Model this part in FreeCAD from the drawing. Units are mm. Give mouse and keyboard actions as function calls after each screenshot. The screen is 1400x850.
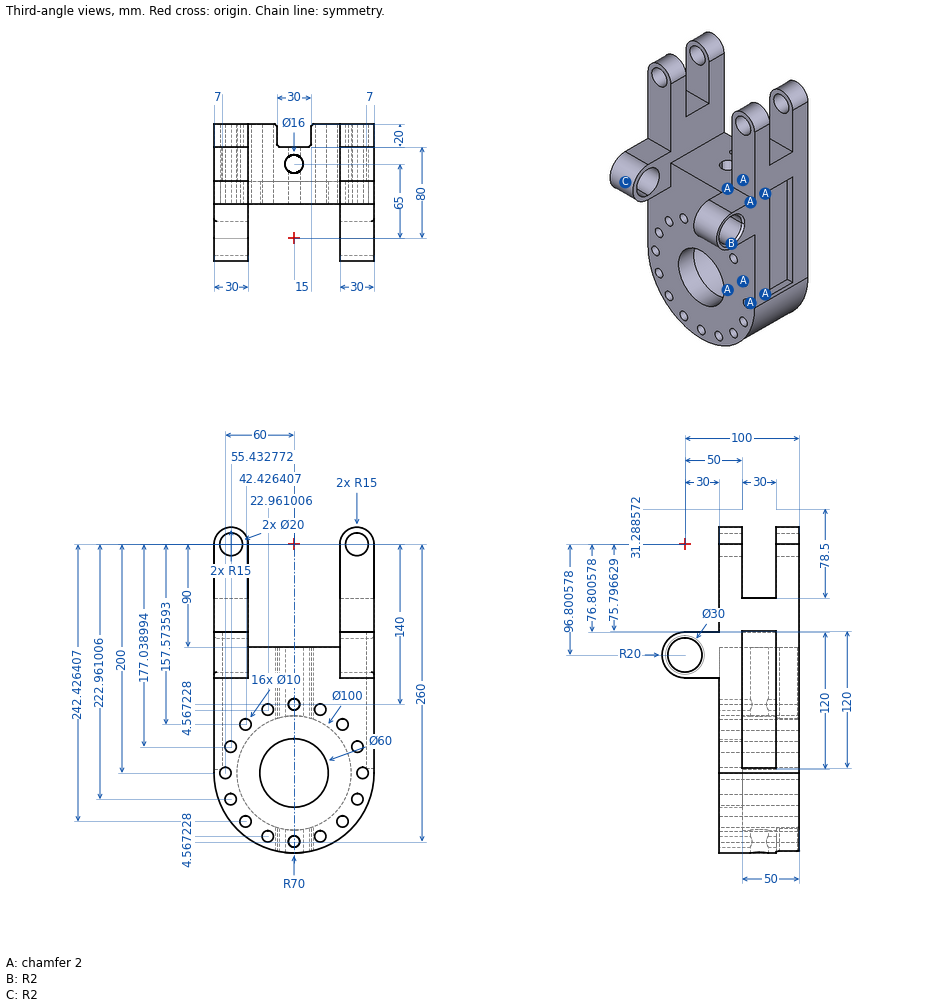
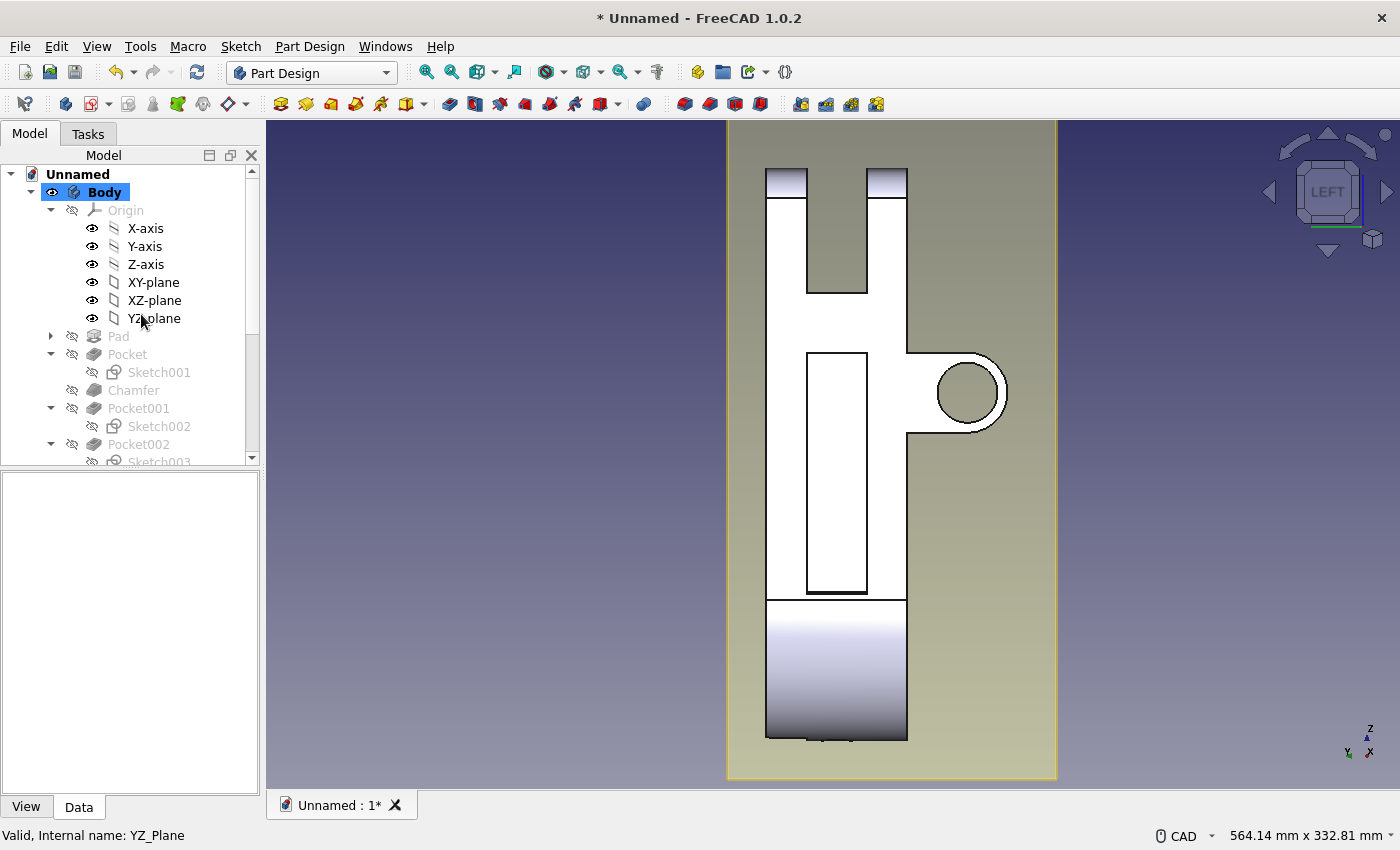
scroll(101, 314, down, 6)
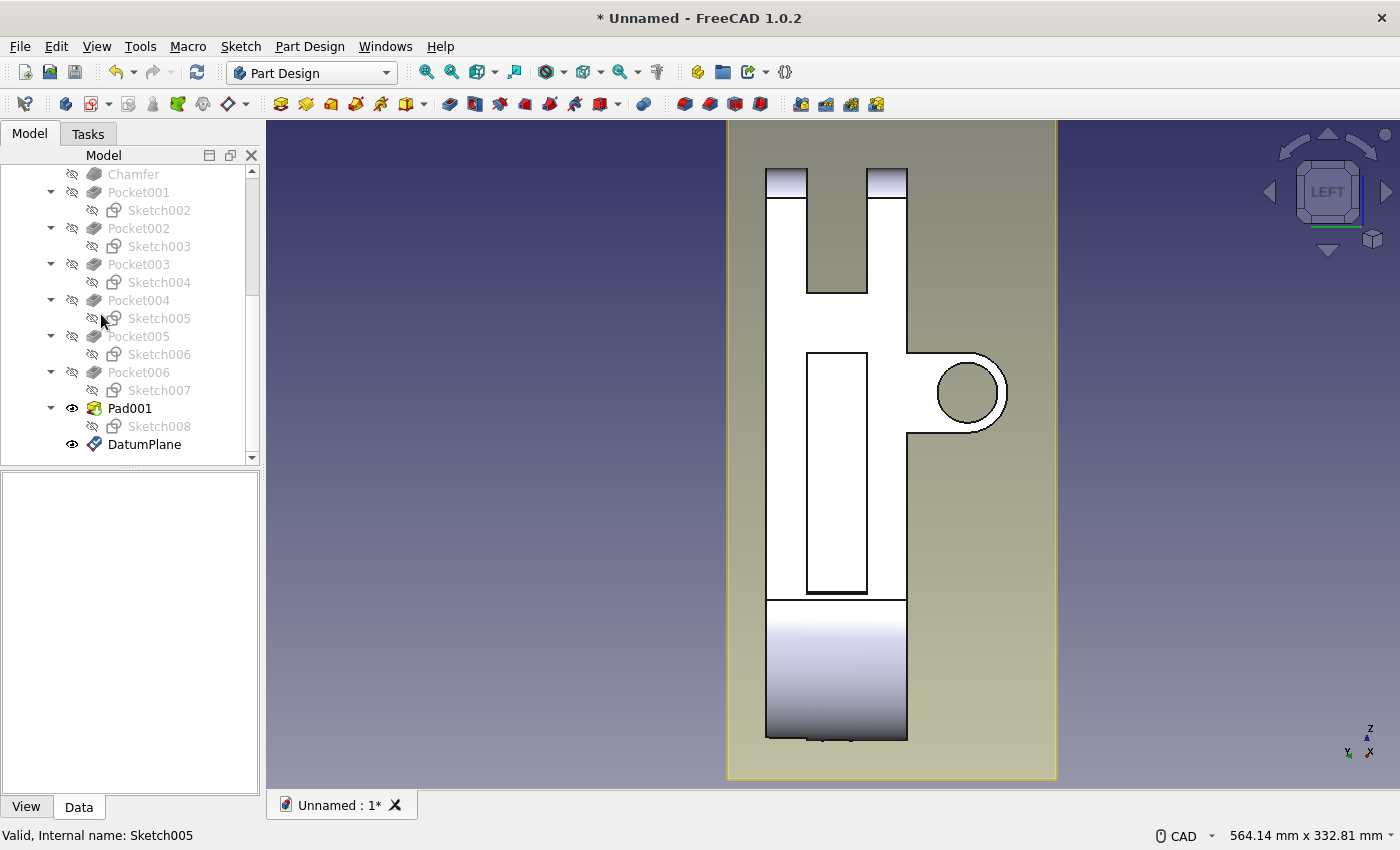
click(117, 444)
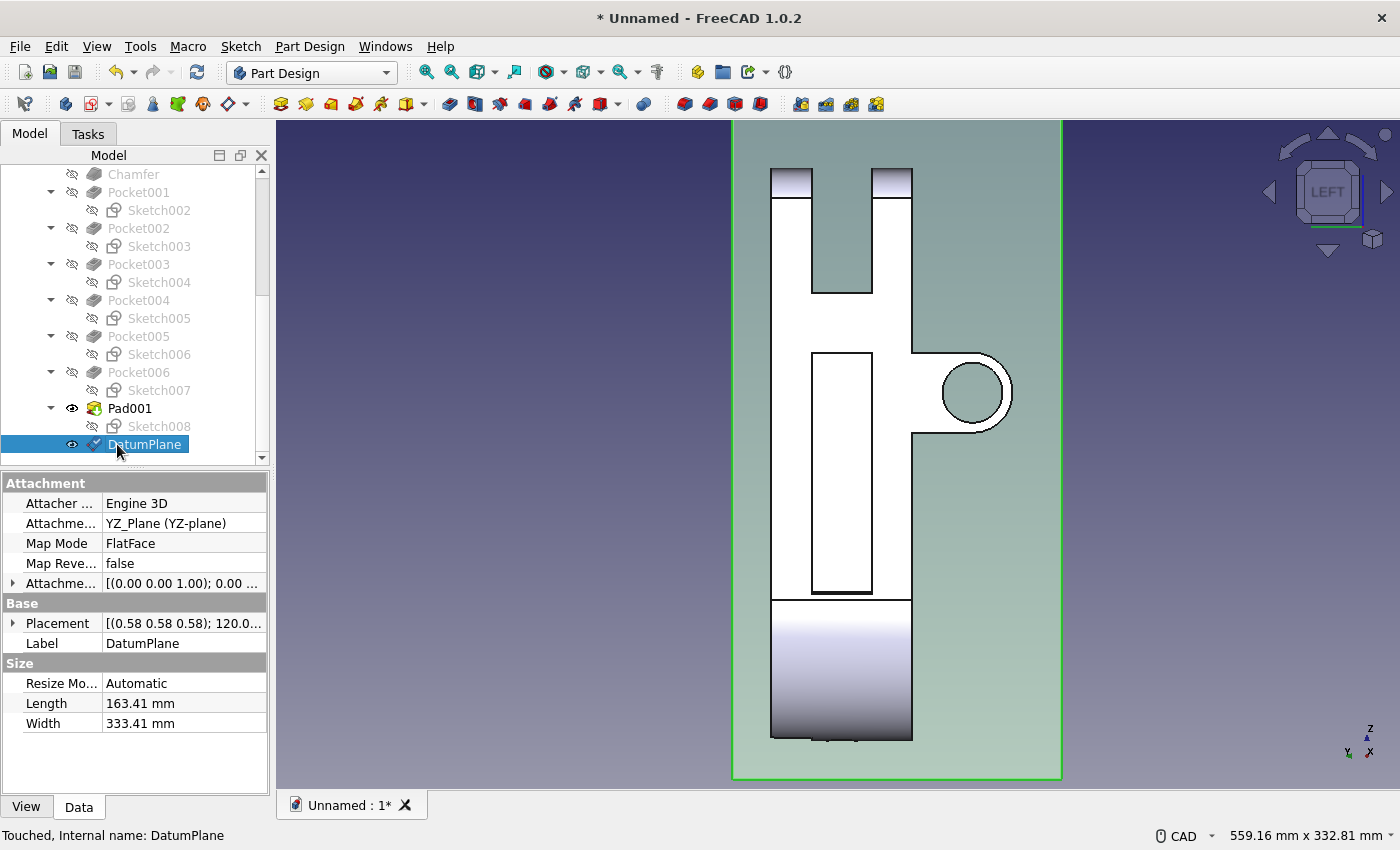
click(90, 104)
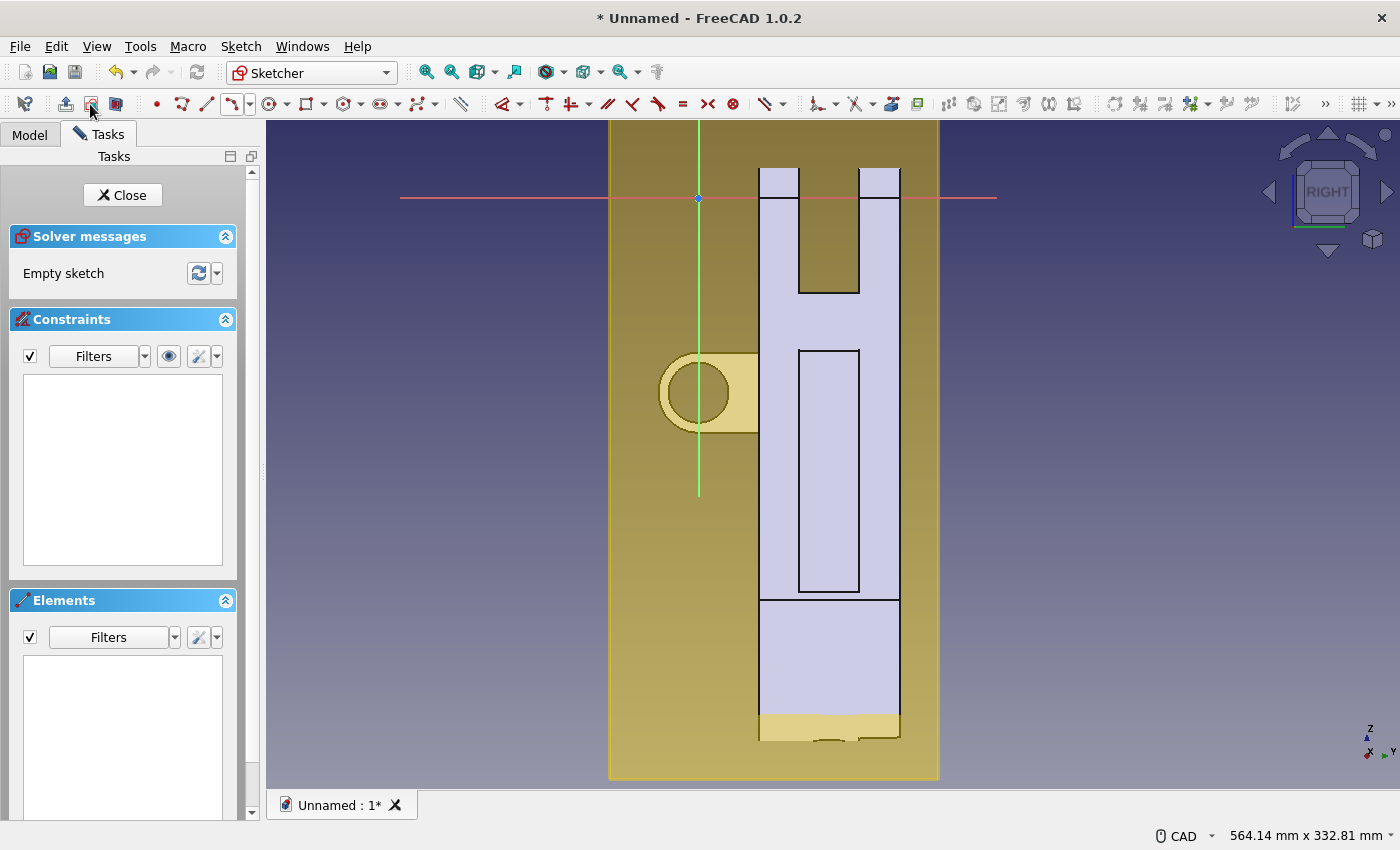
key(q)
key(s)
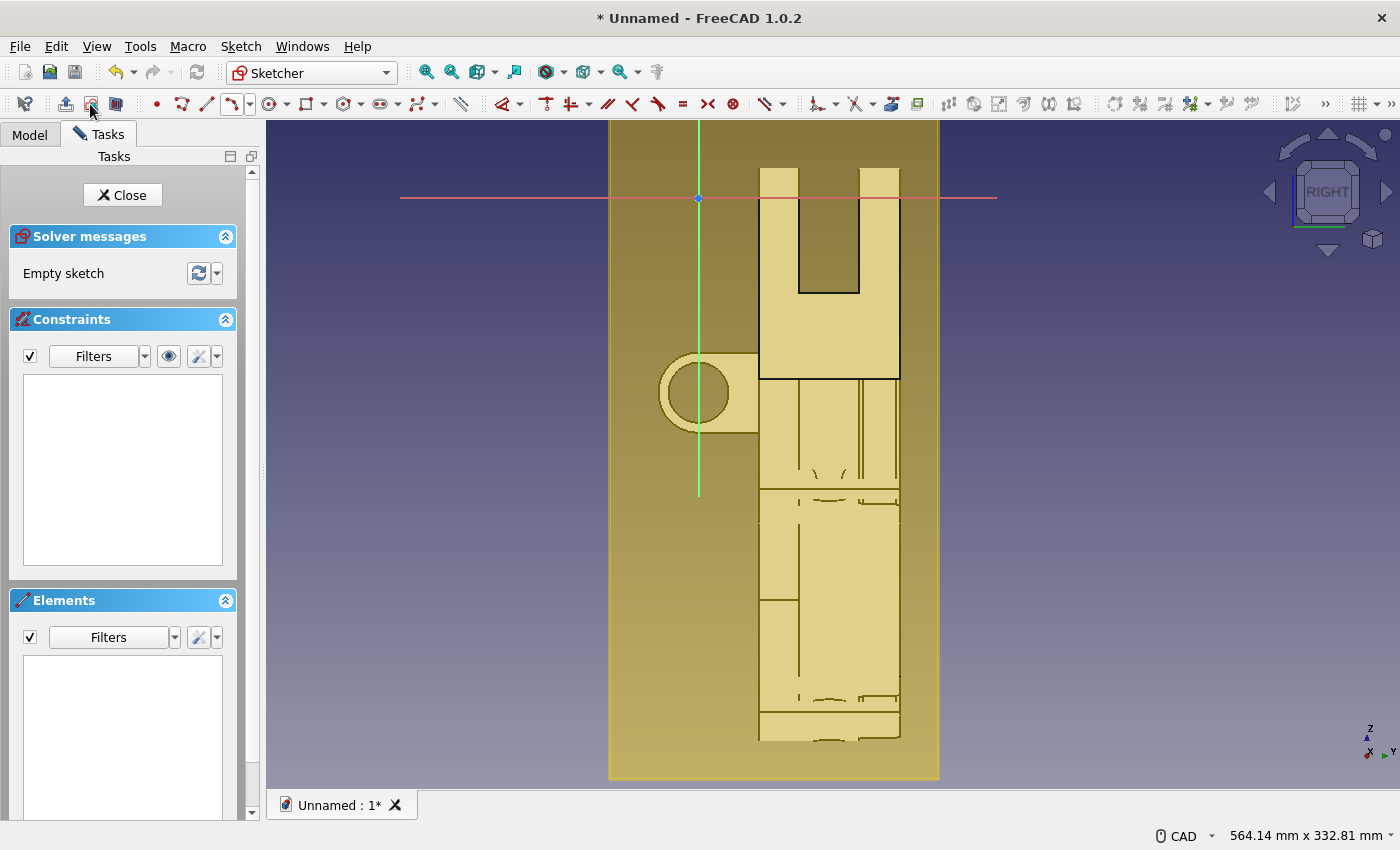
scroll(641, 148, up, 3)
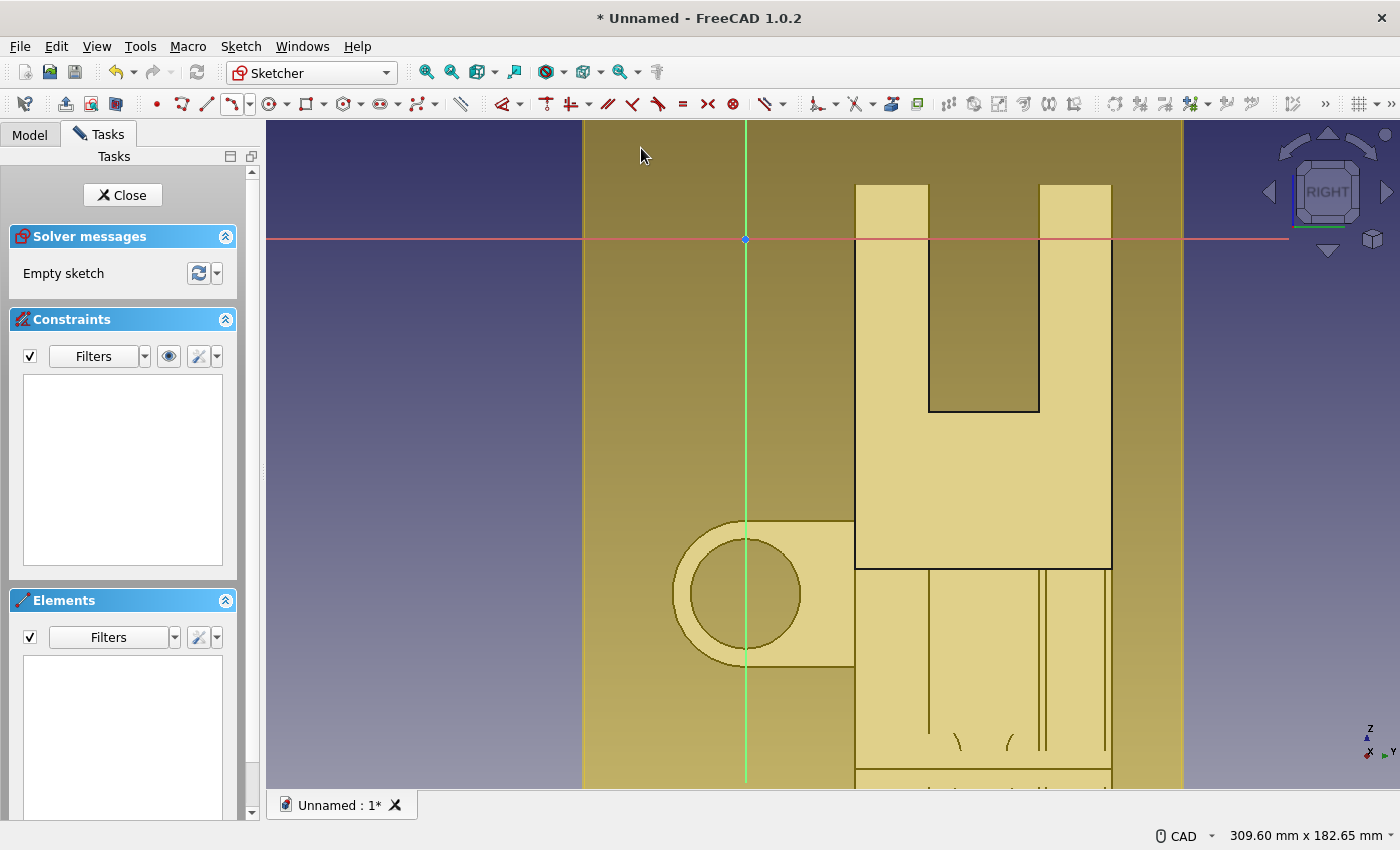
click(182, 104)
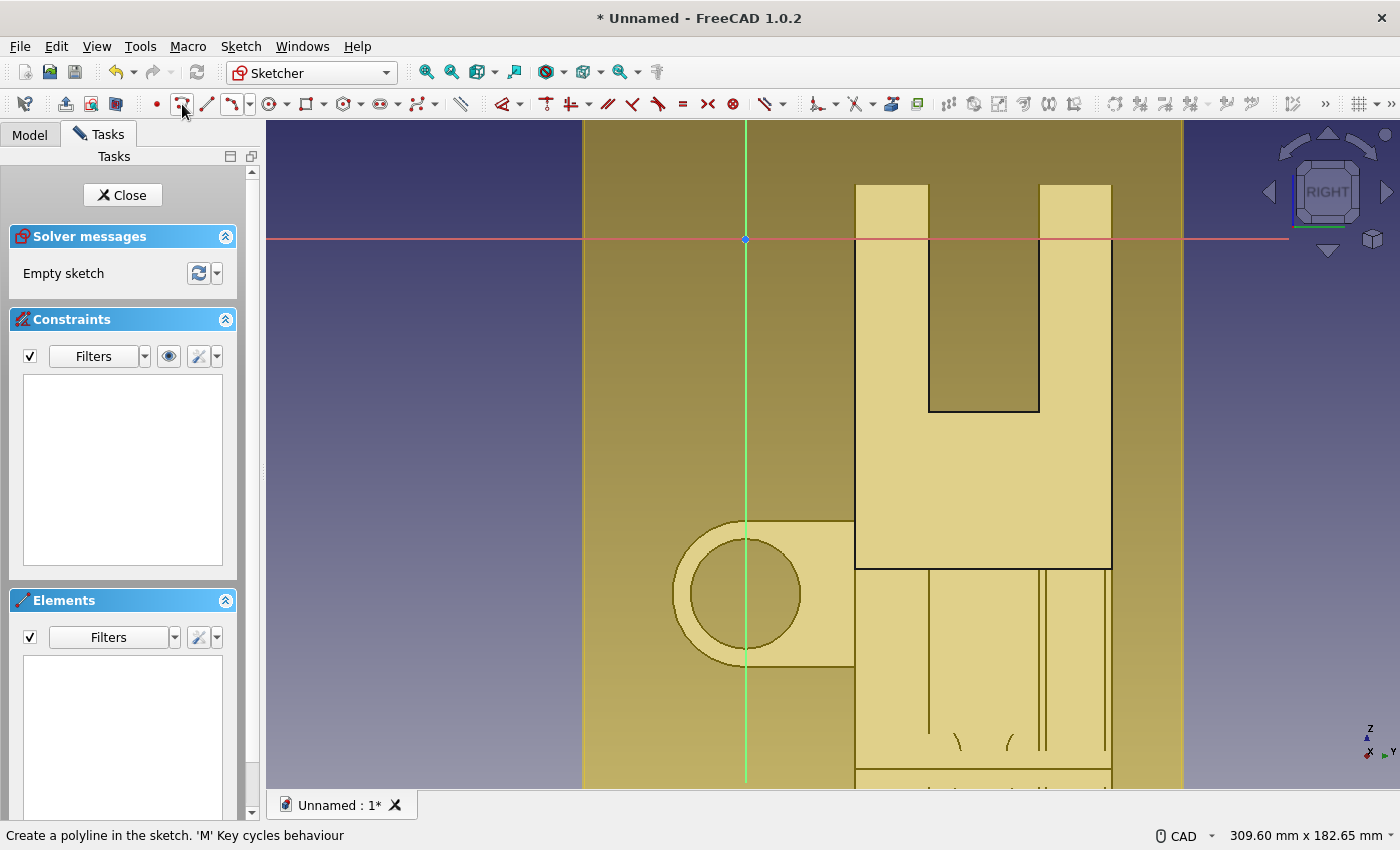
click(746, 667)
click(855, 667)
click(855, 521)
click(746, 521)
right_click(746, 521)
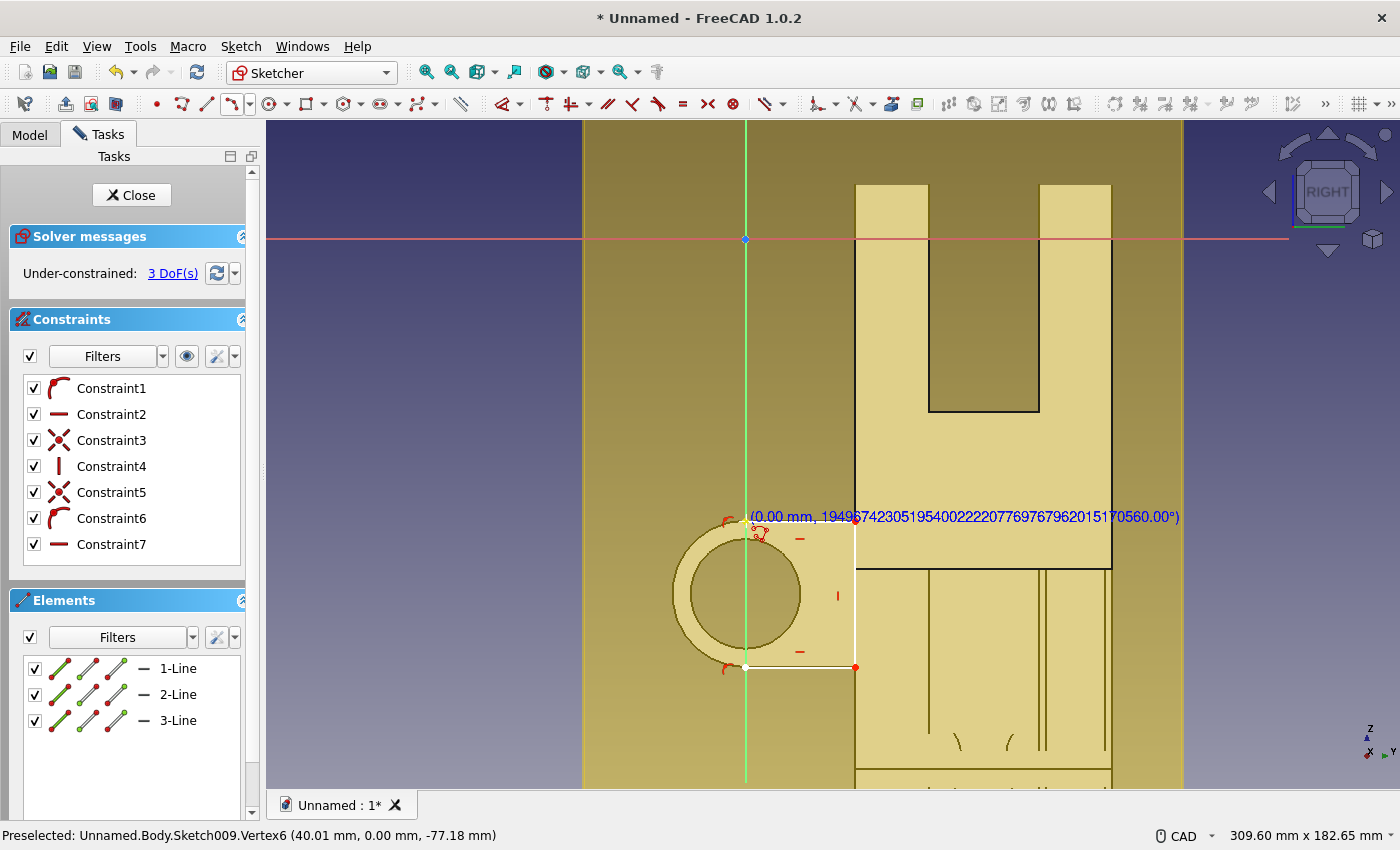
key(g)
key(3)
key(a)